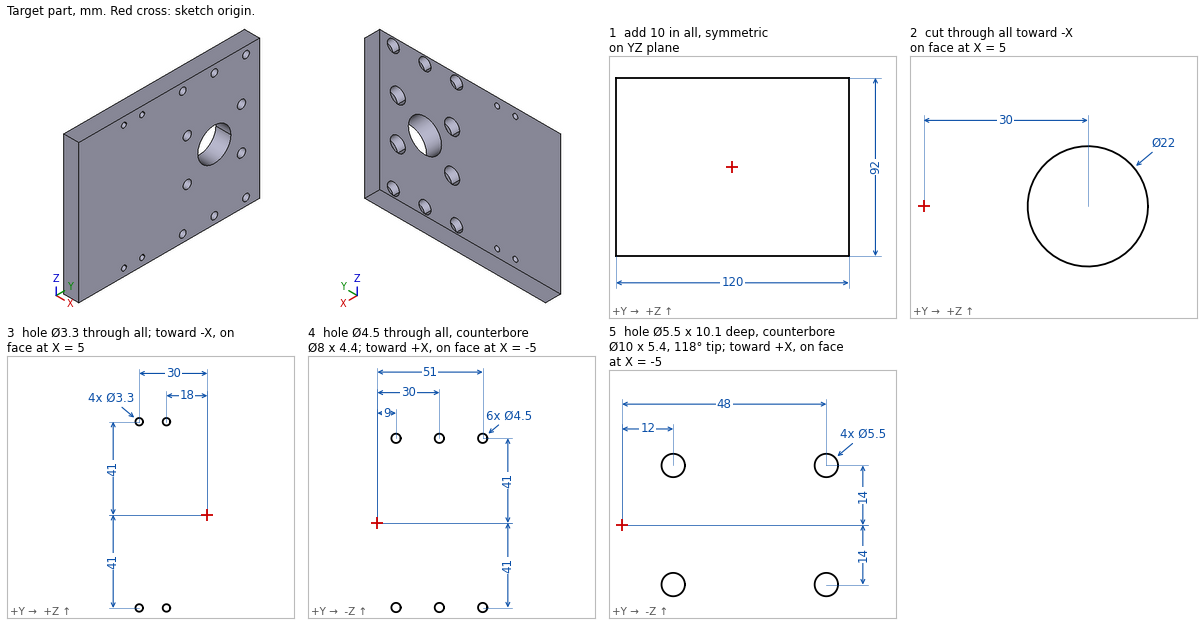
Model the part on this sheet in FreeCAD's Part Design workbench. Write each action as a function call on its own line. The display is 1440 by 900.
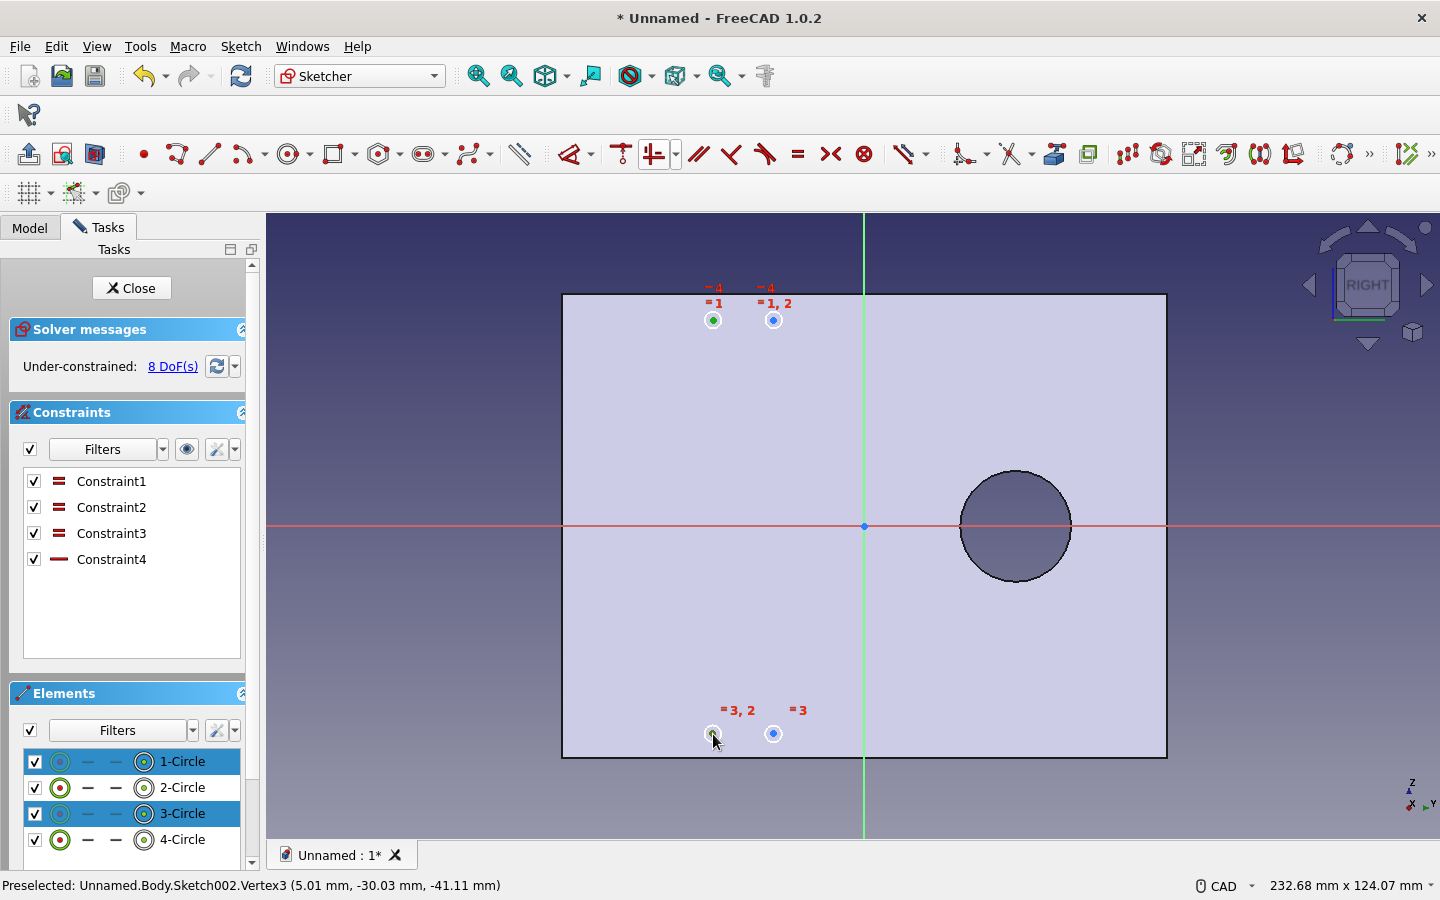
click(676, 154)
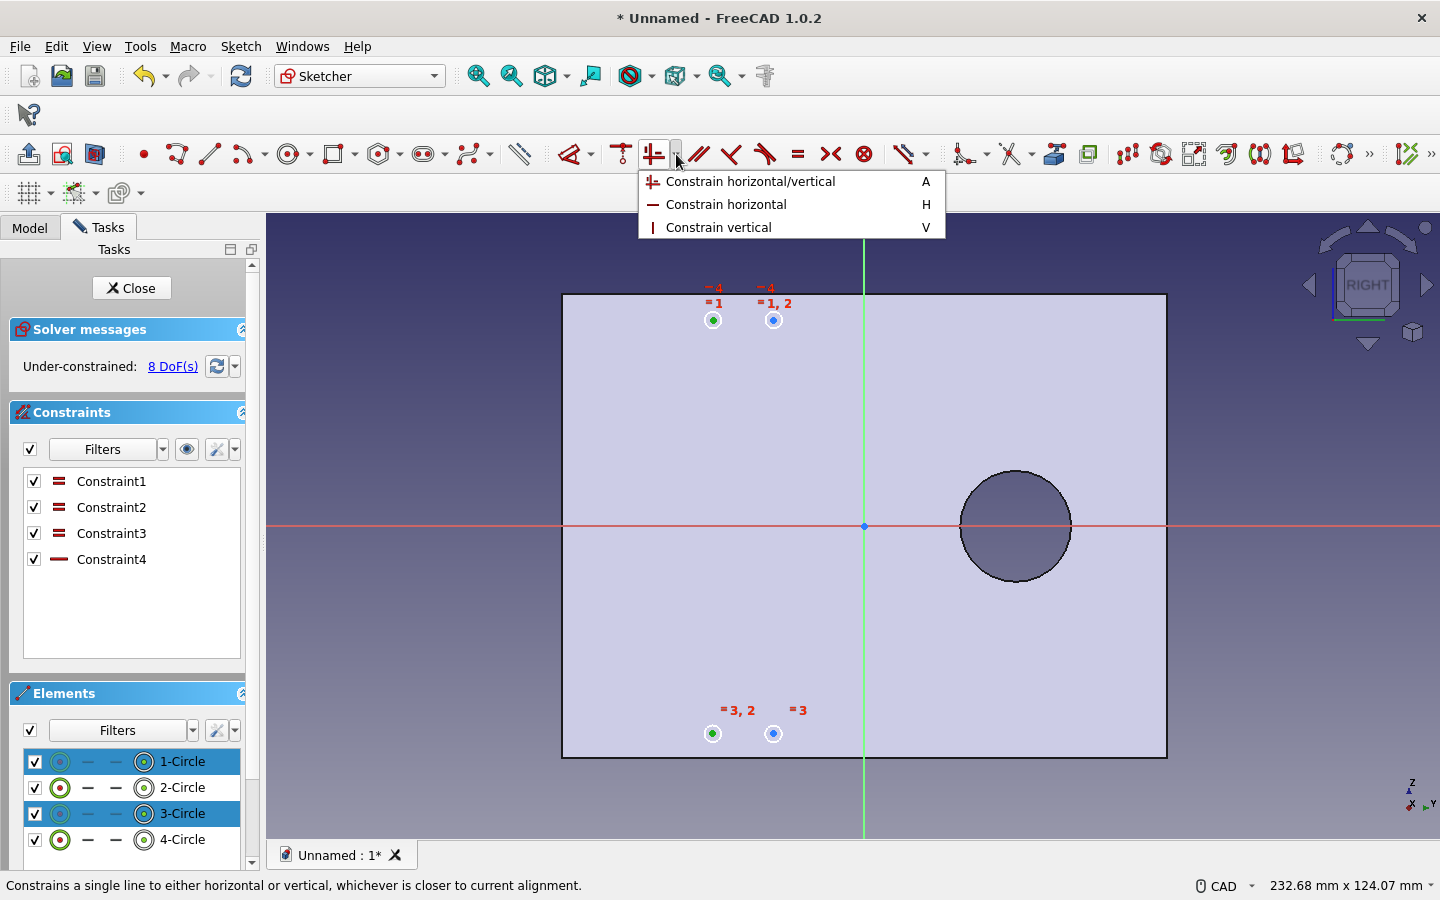
click(792, 228)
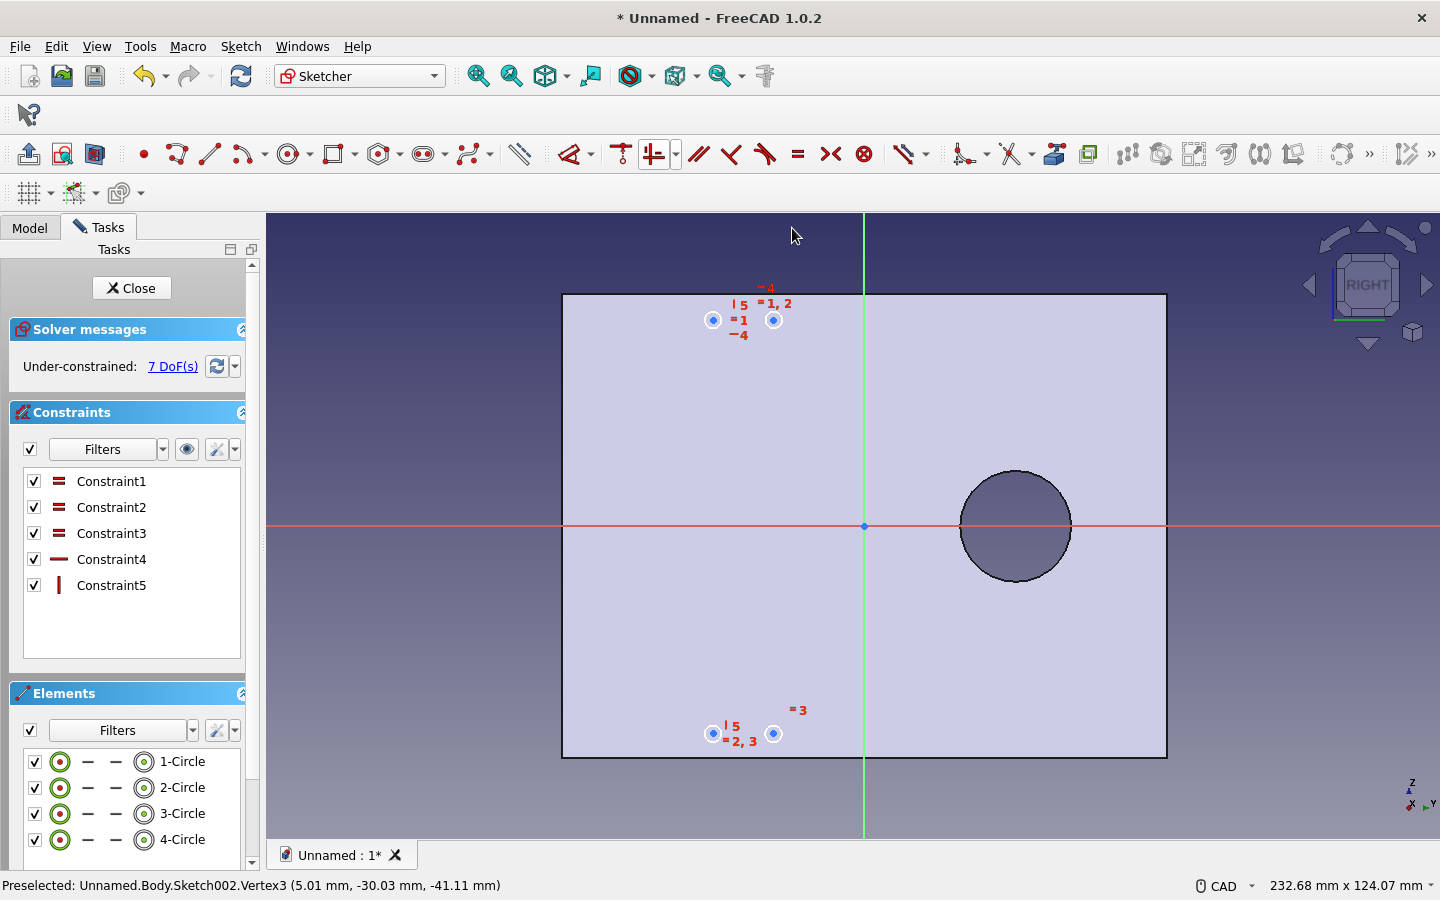
click(774, 320)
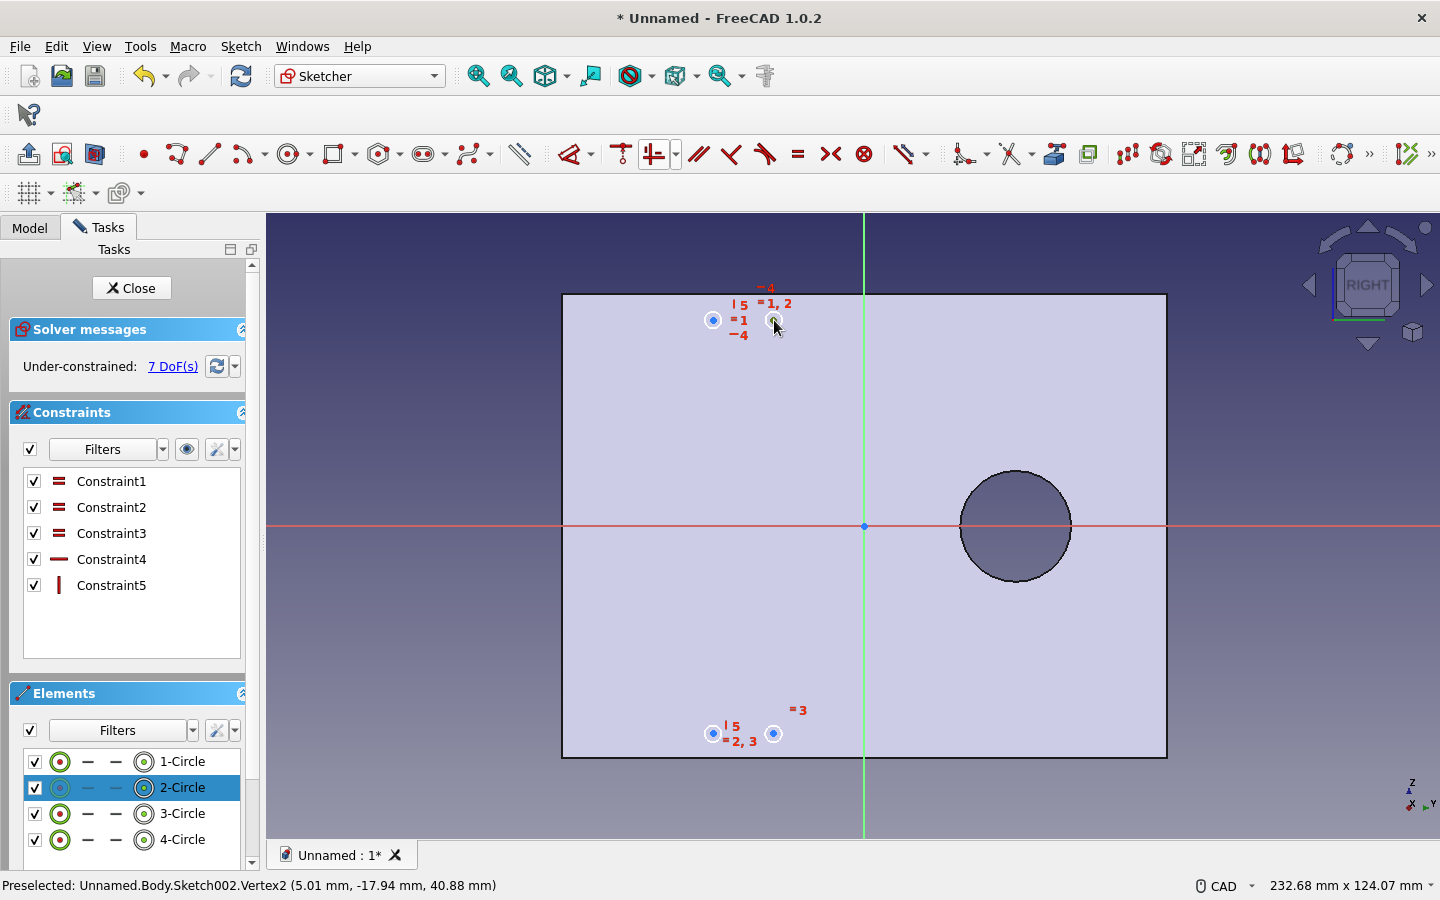
click(774, 734)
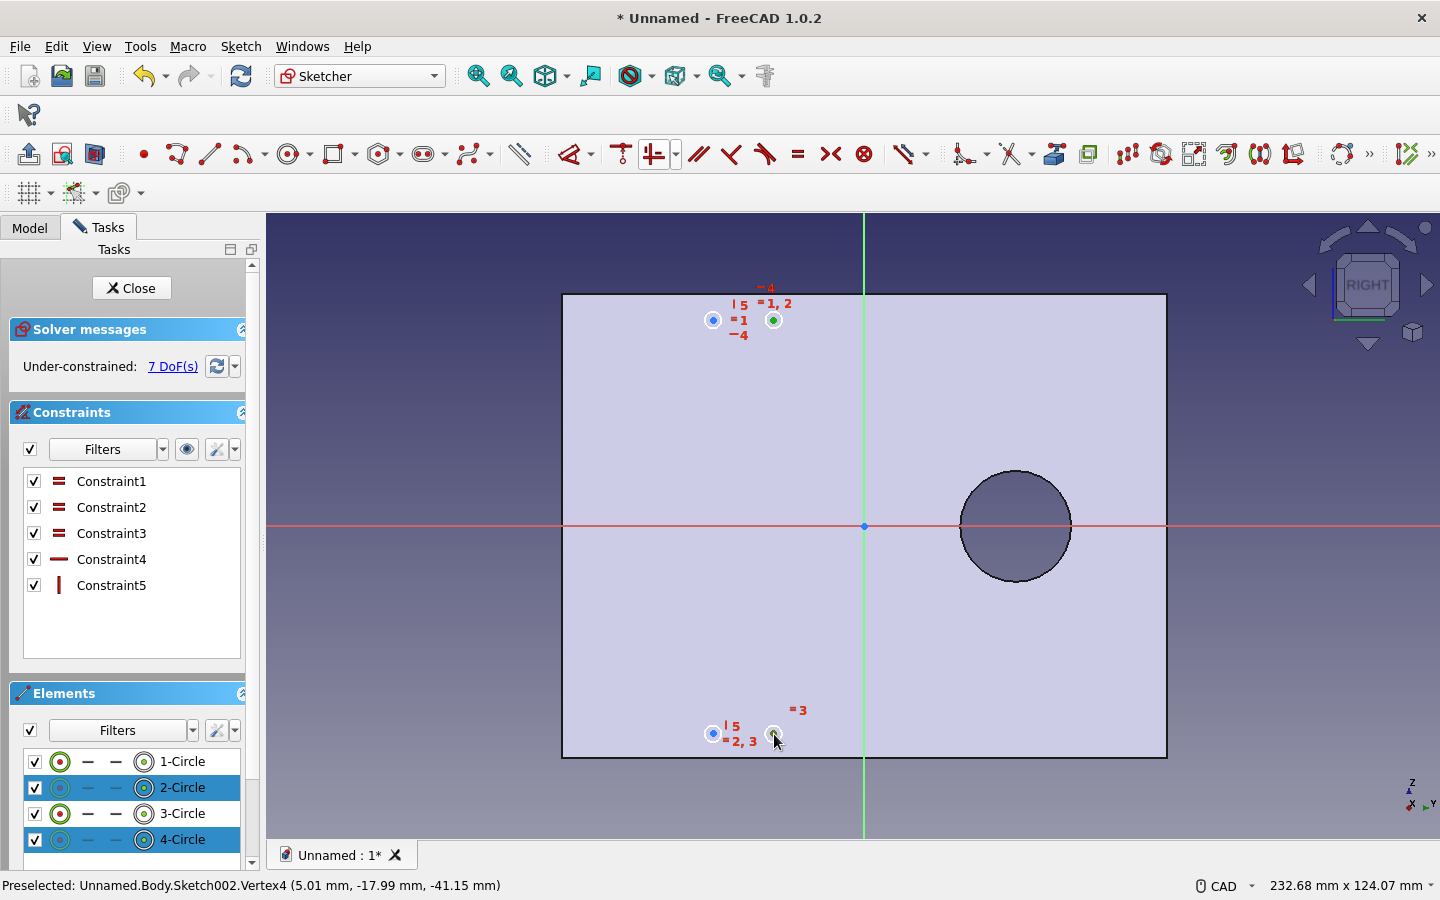
key(v)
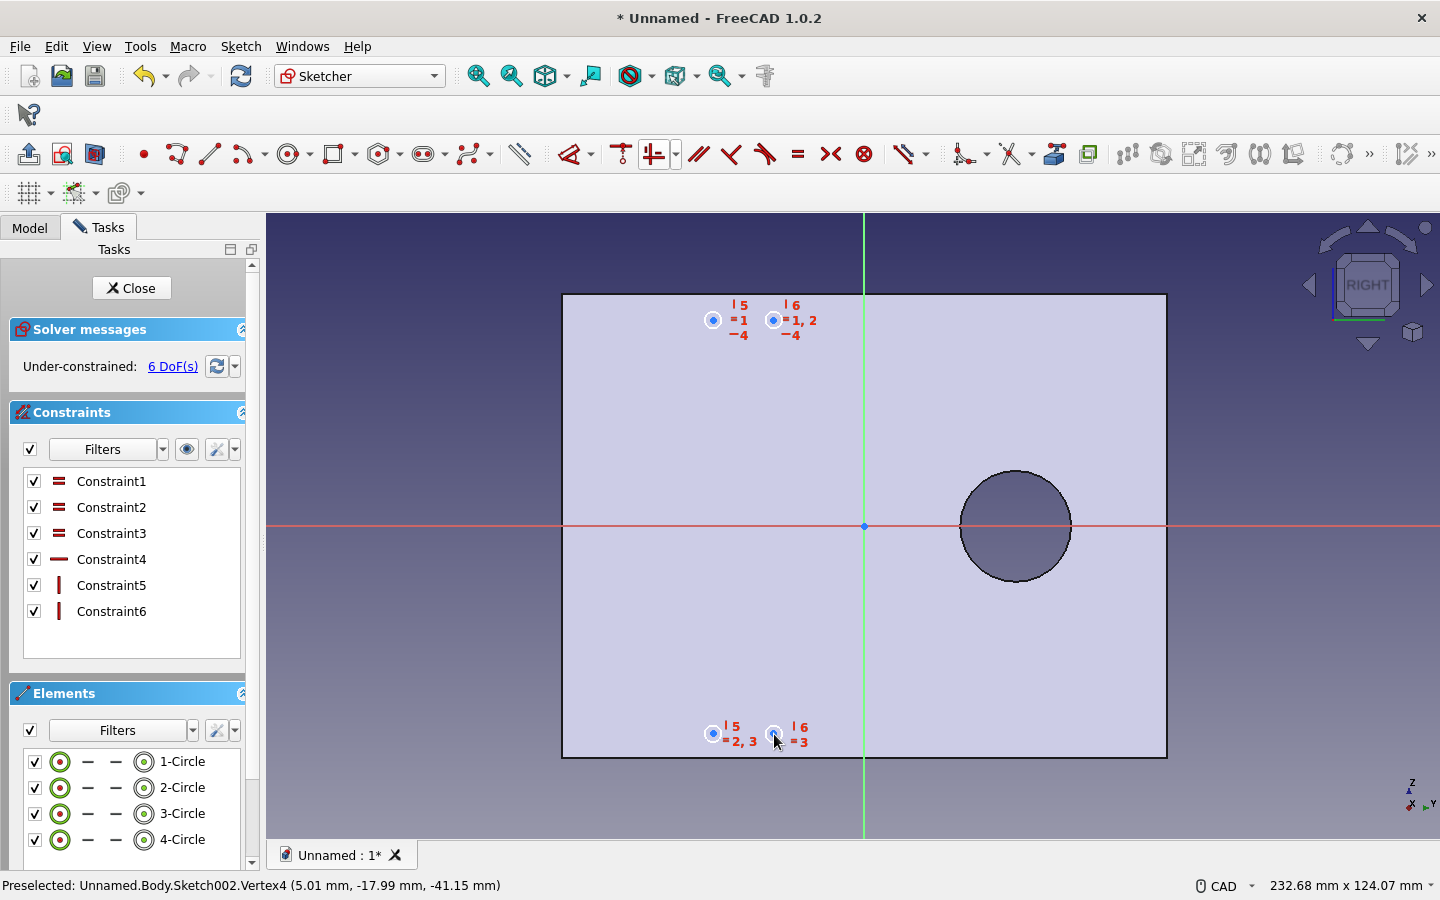
click(713, 734)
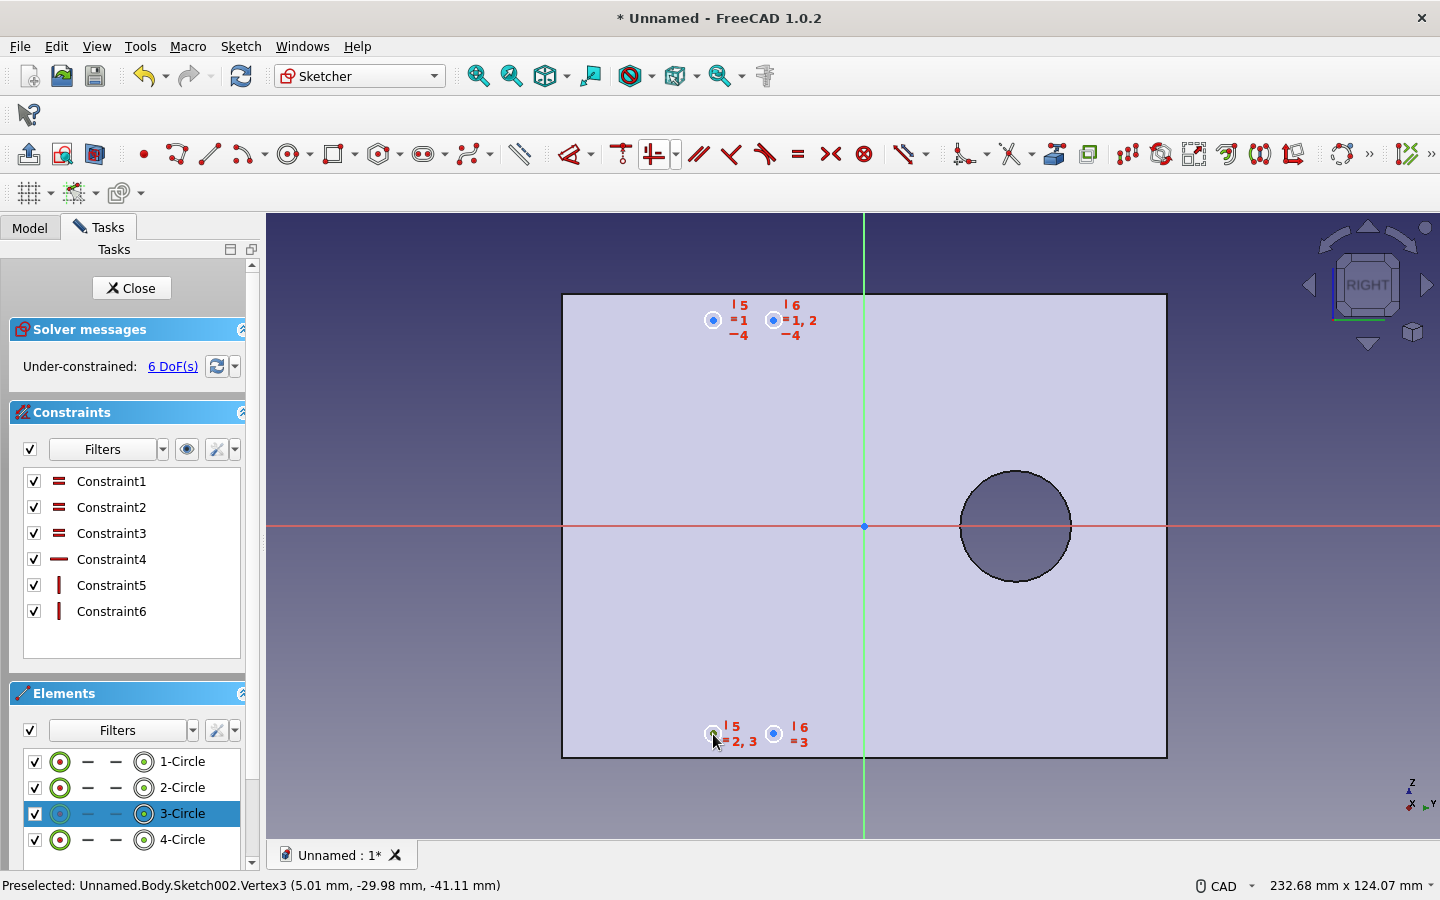
click(774, 734)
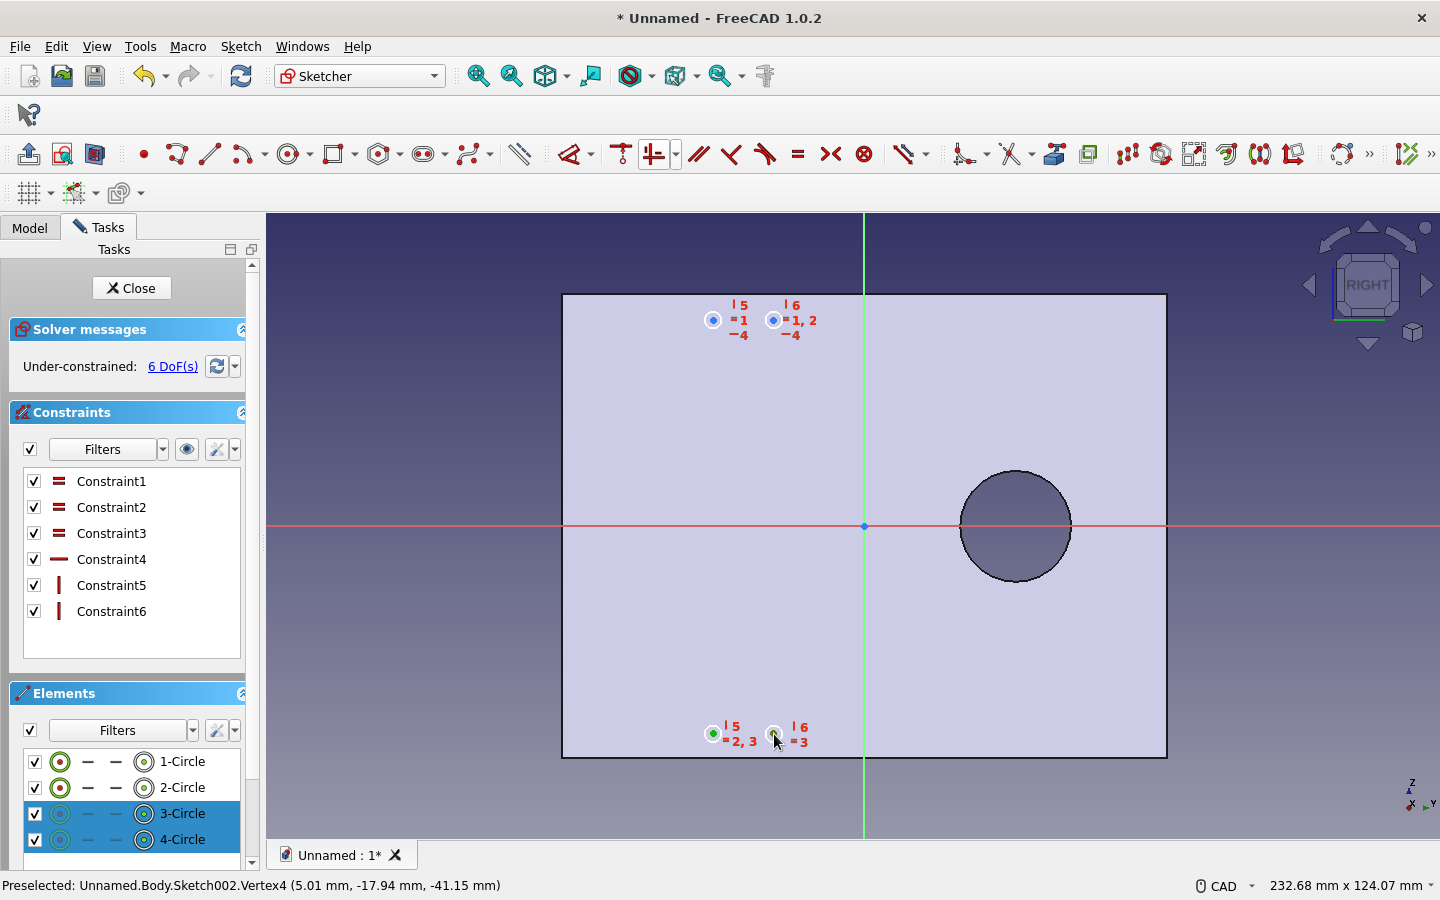
key(h)